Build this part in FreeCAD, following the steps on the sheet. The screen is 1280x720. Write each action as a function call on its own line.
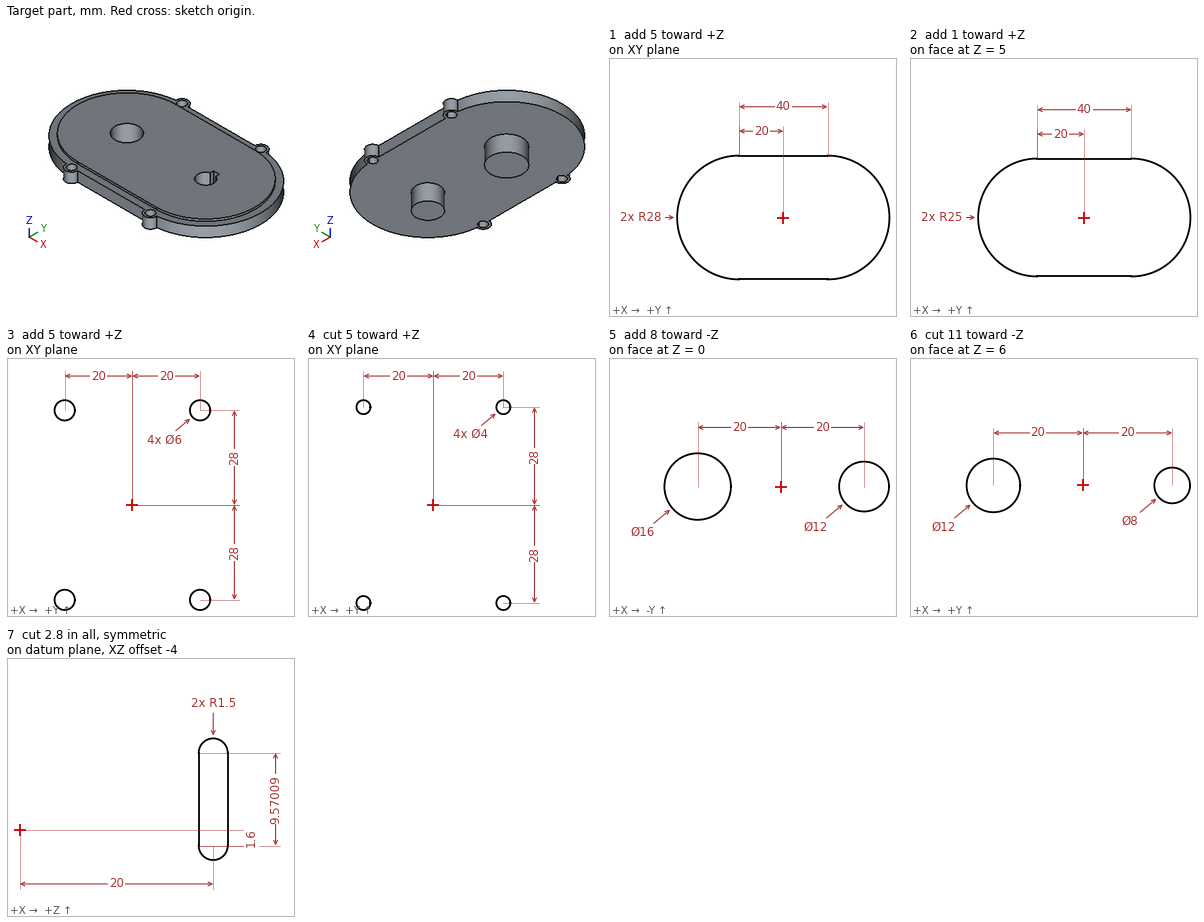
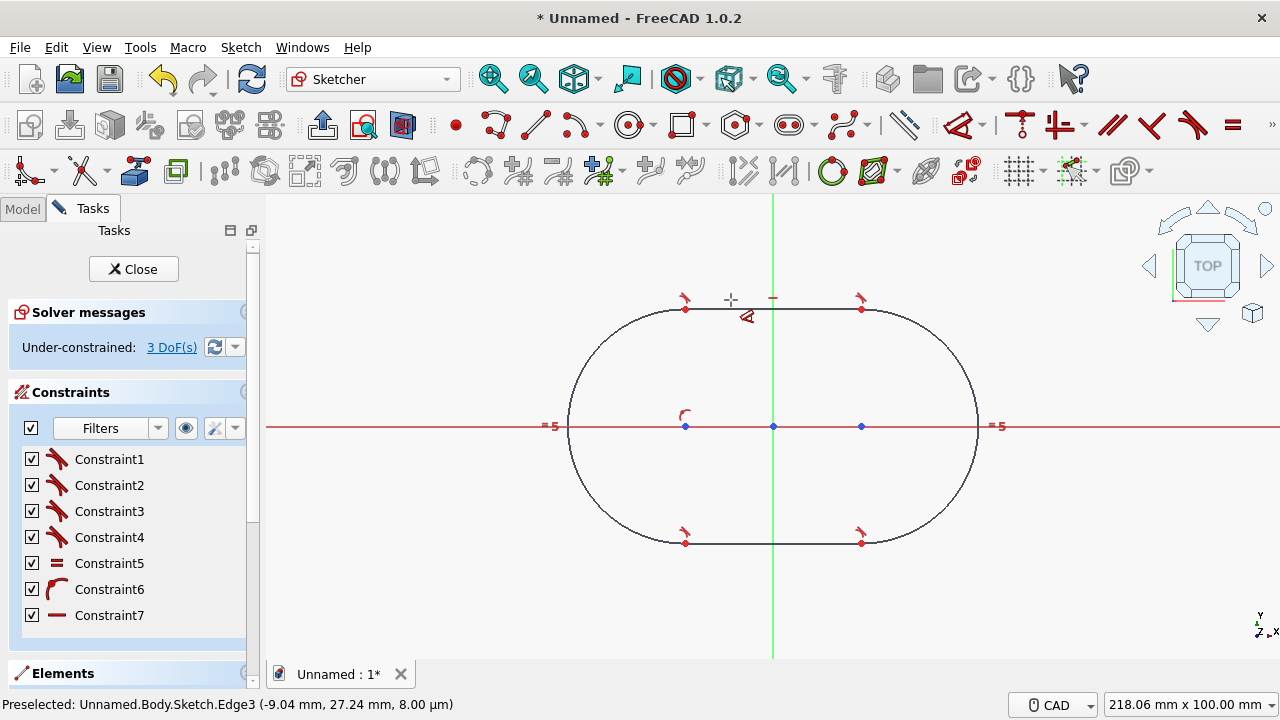
click(590, 358)
click(564, 339)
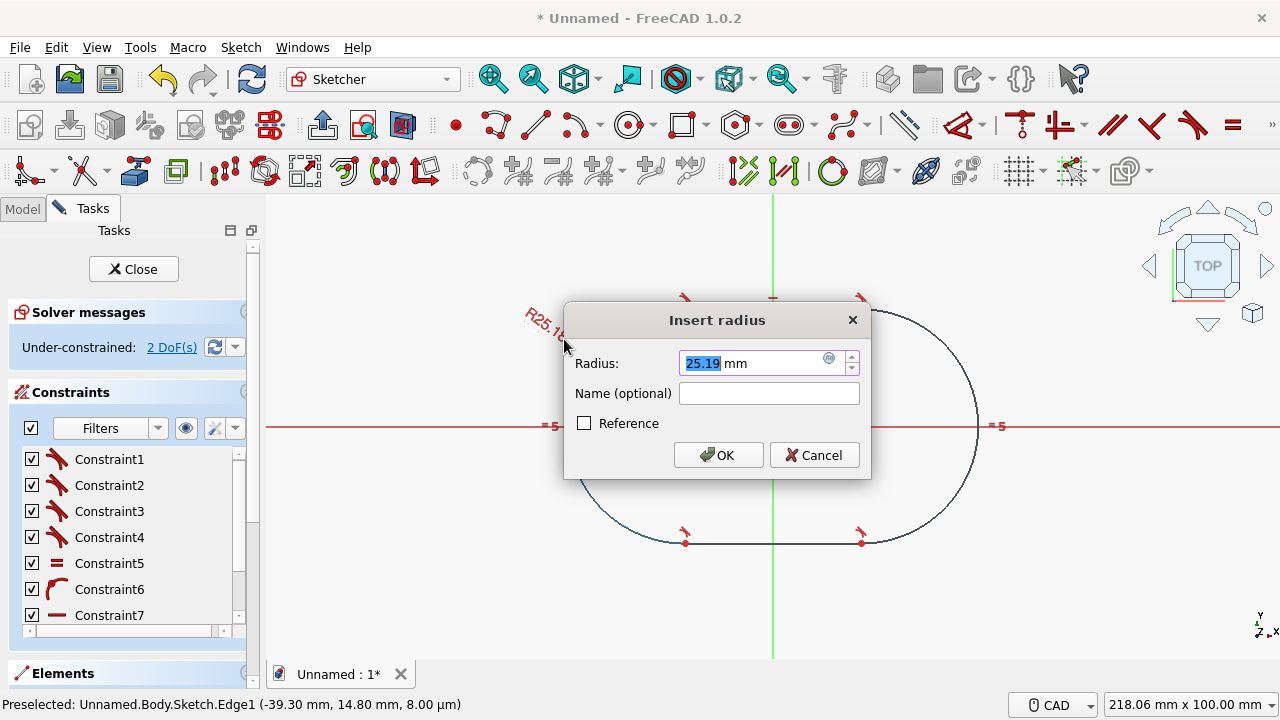
text(28)
key(Return)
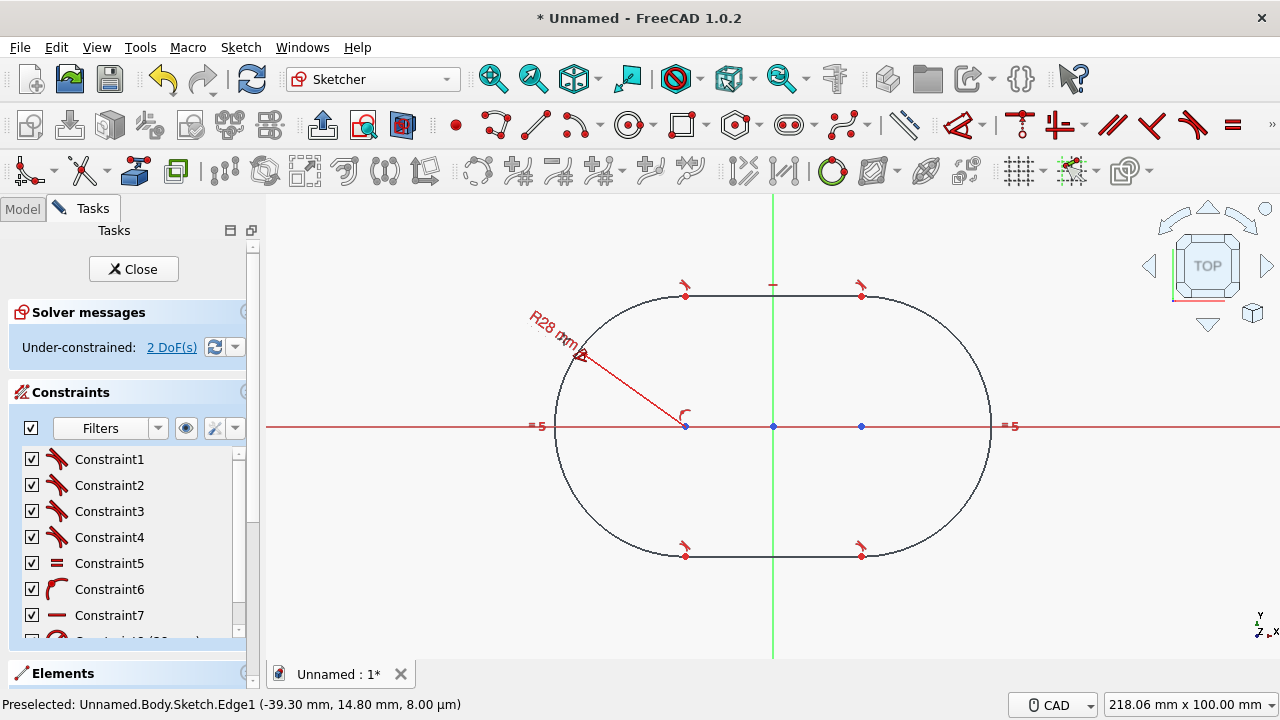
click(738, 296)
click(733, 262)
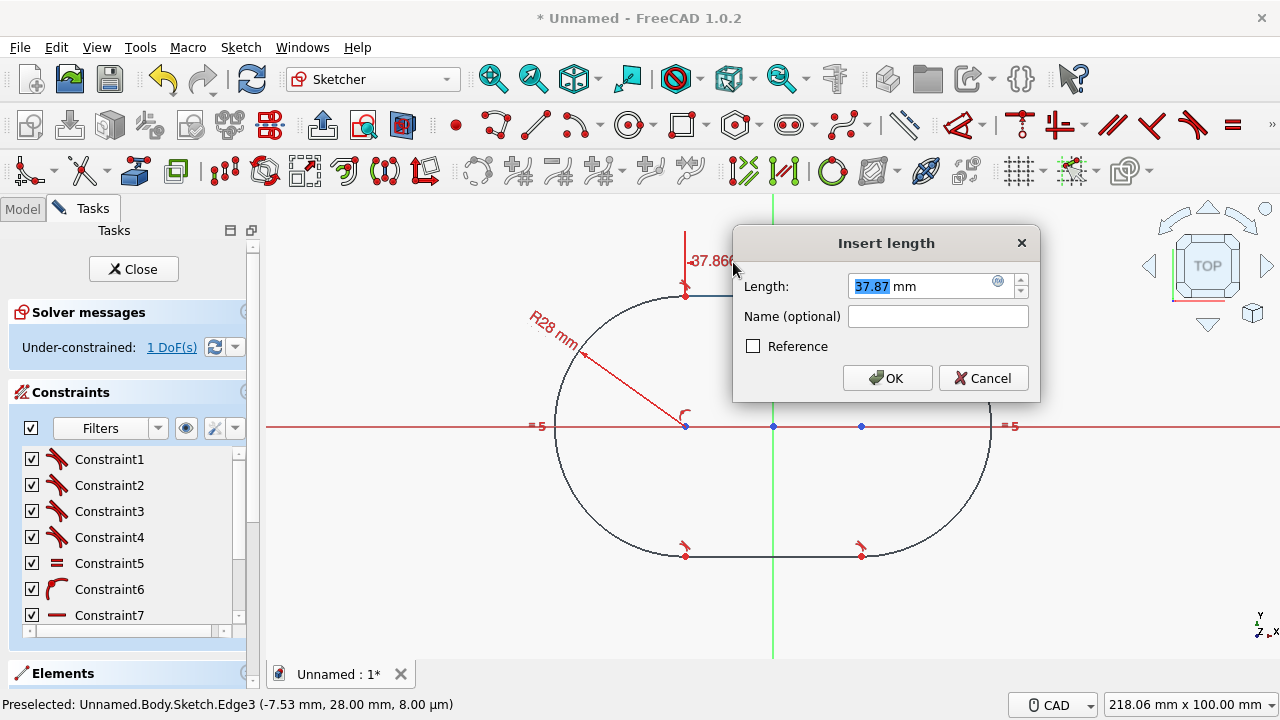
text(40)
key(Return)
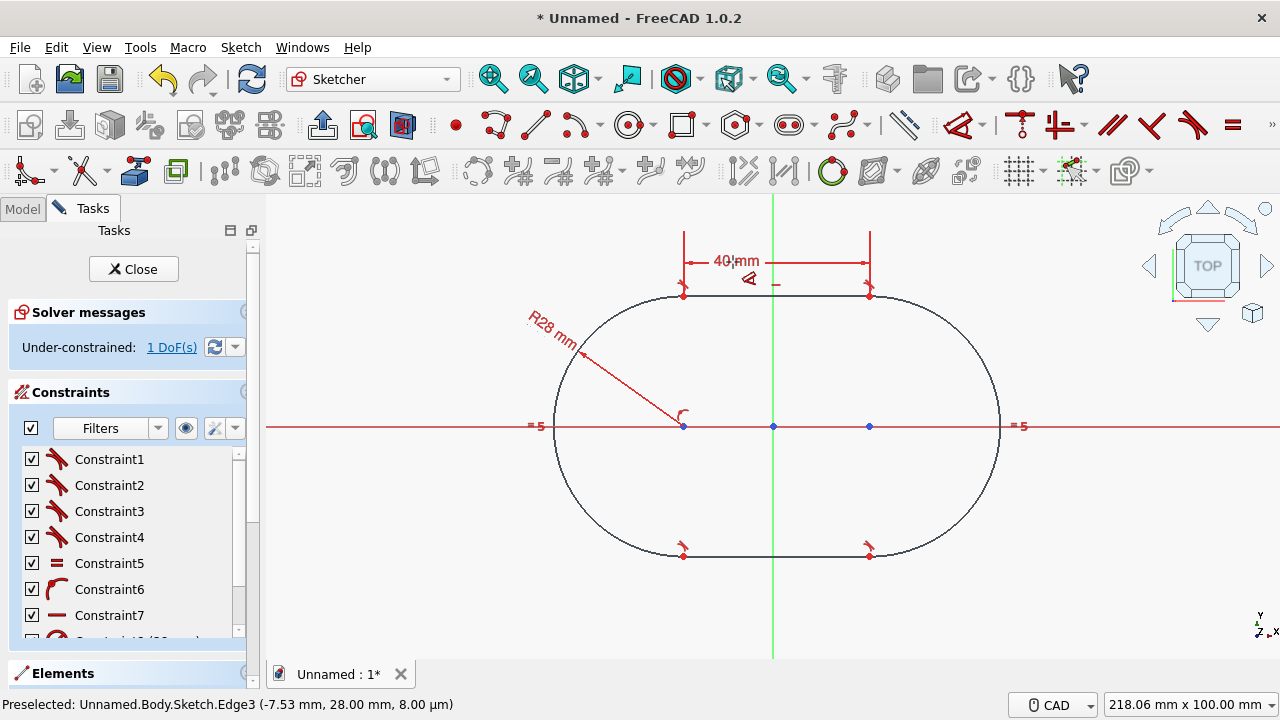
click(684, 296)
click(728, 460)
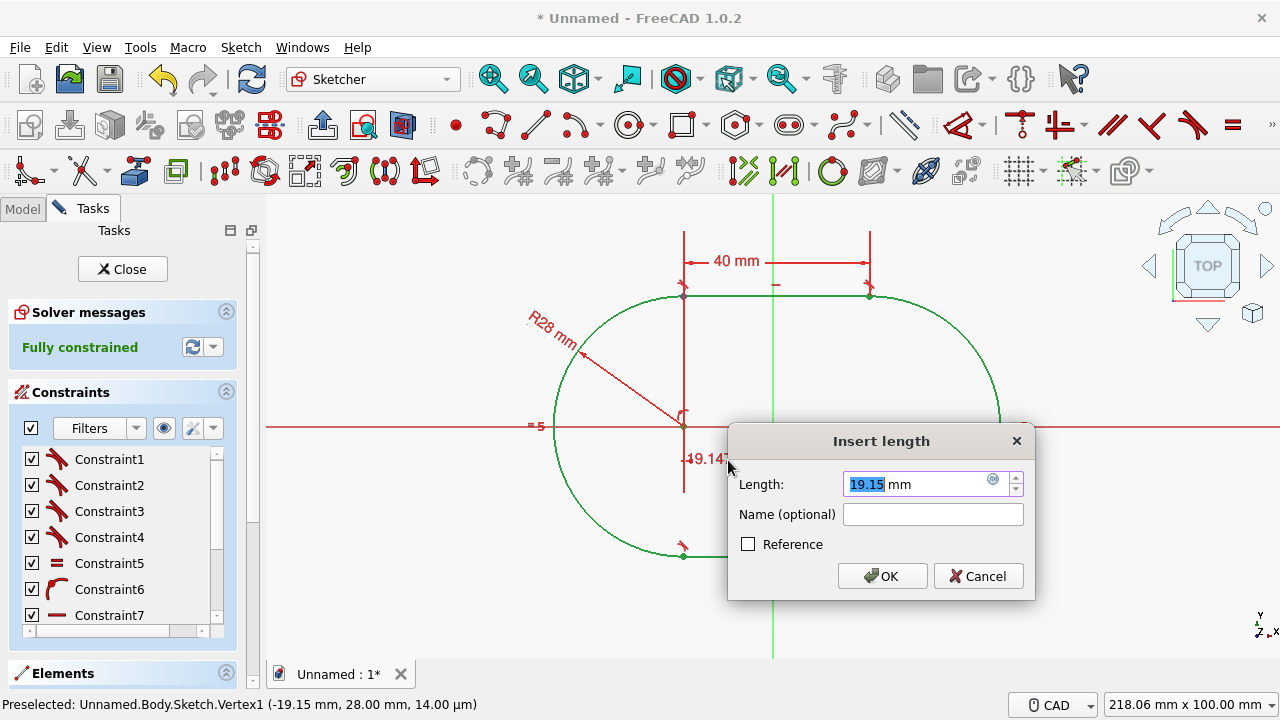
text(20)
key(Return)
key(Escape)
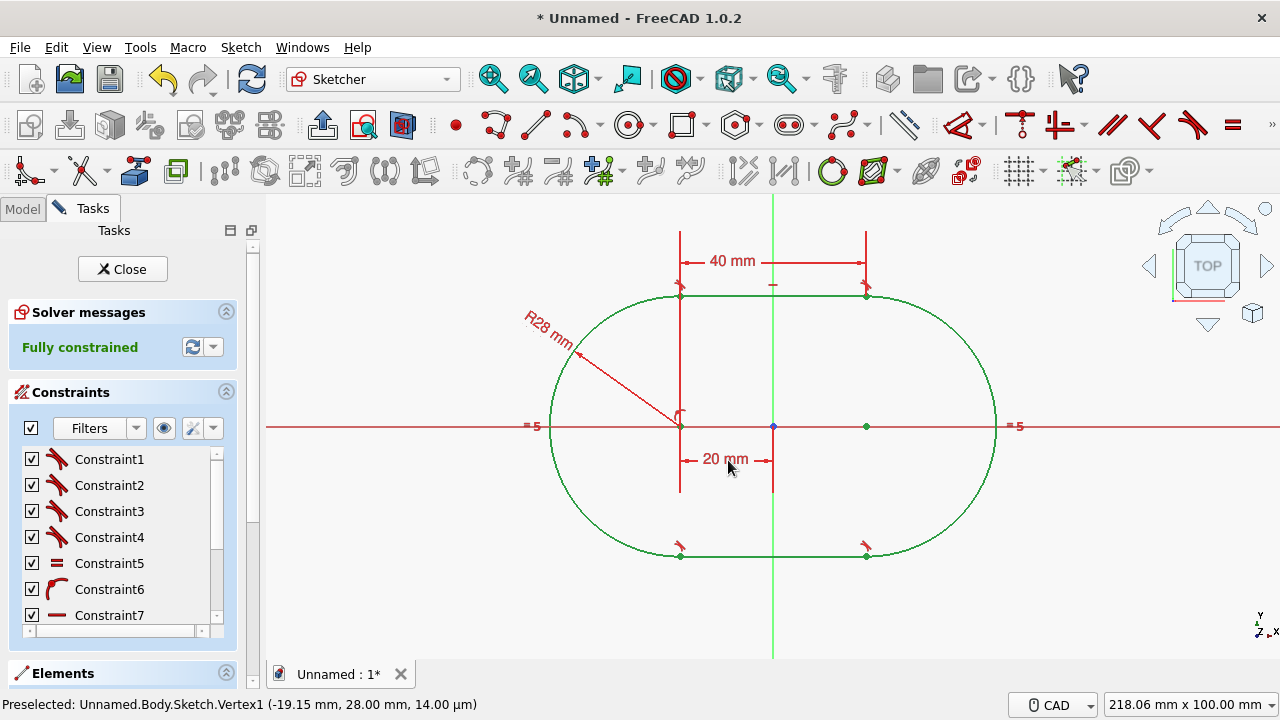
click(123, 269)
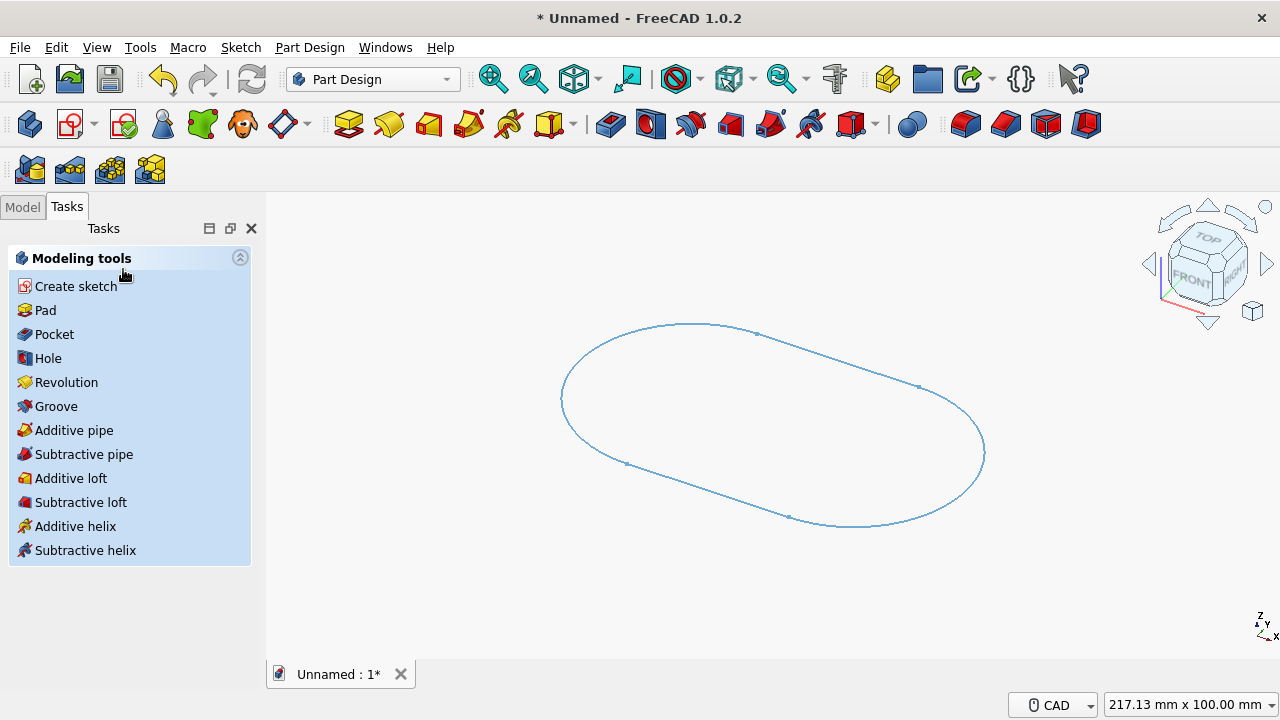
click(350, 124)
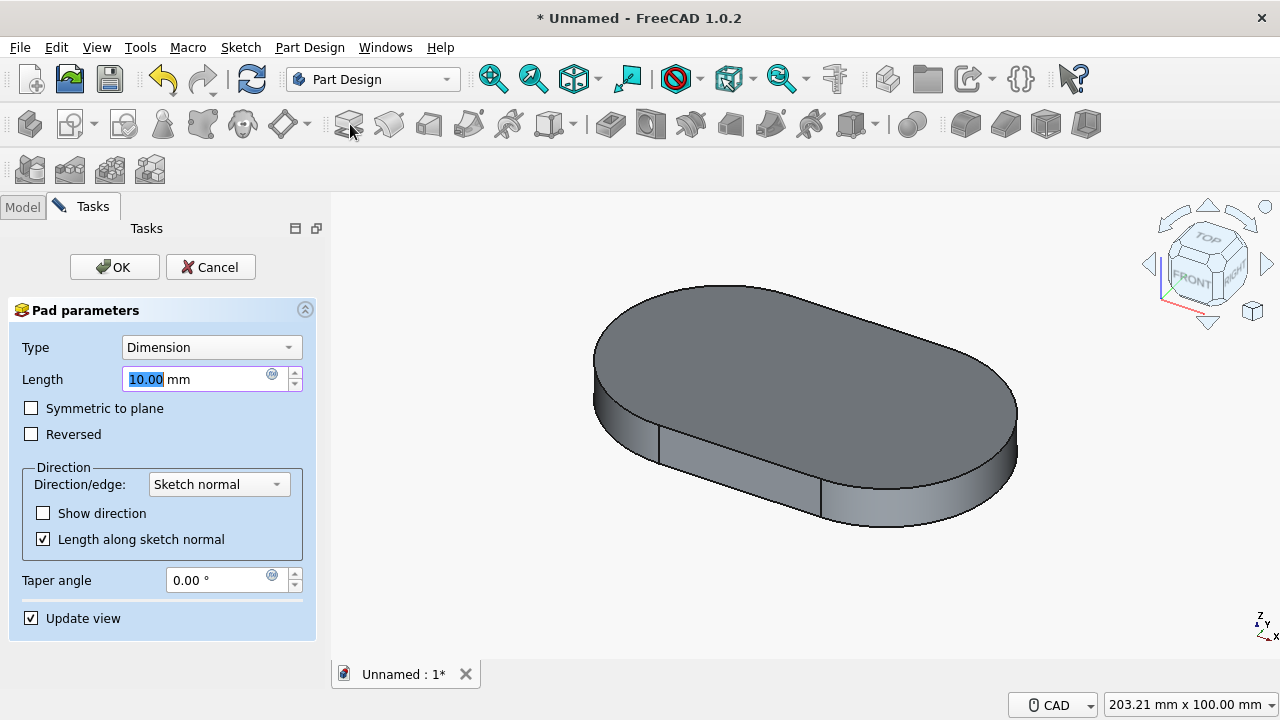
text(5)
key(Tab)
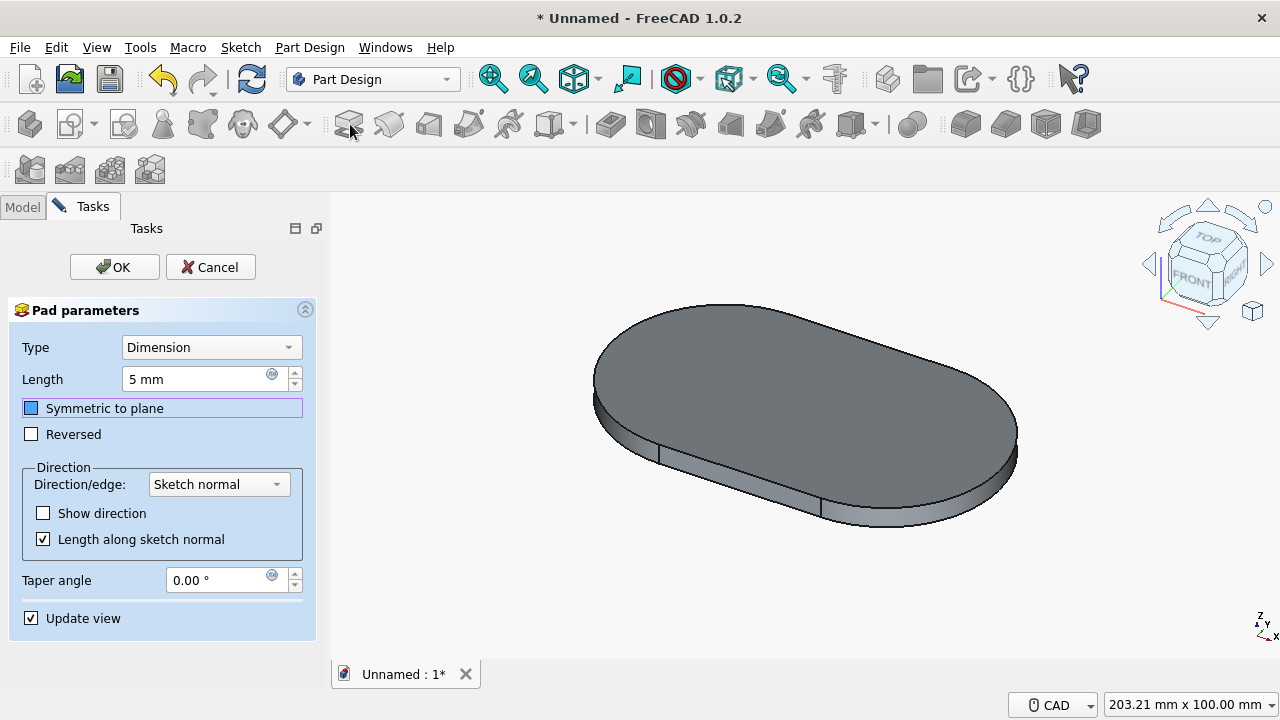
click(115, 267)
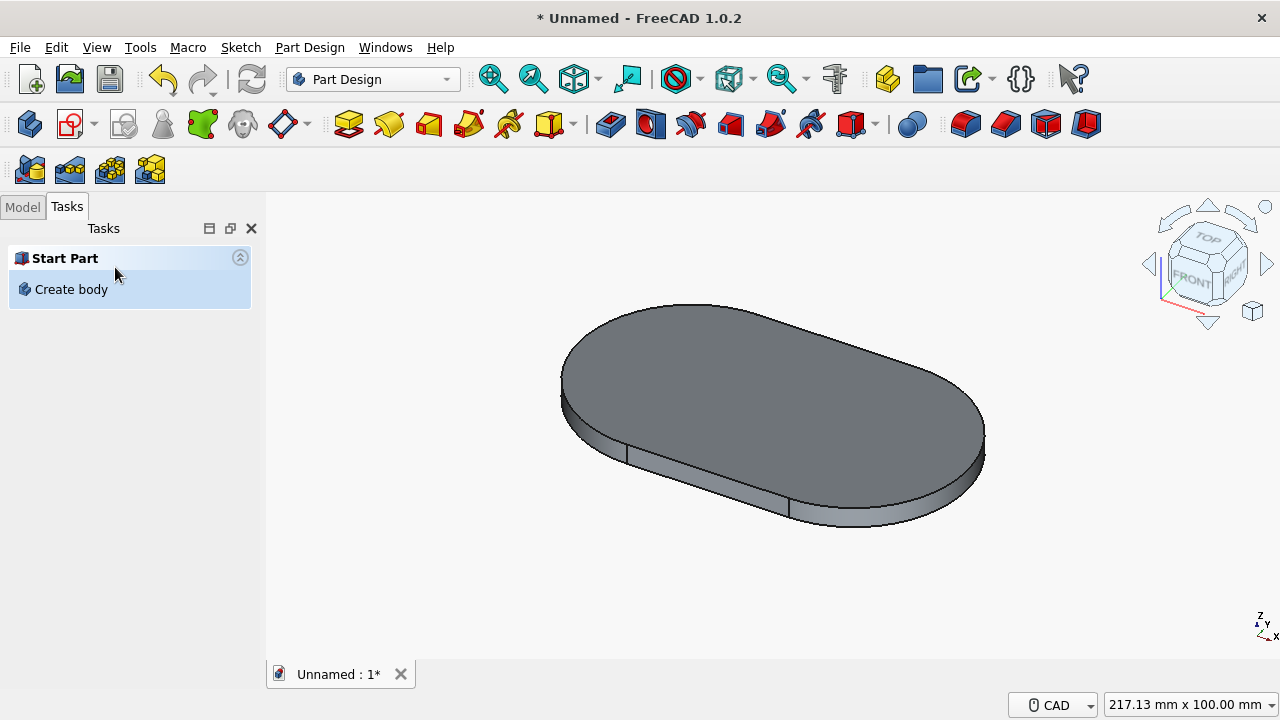
click(828, 424)